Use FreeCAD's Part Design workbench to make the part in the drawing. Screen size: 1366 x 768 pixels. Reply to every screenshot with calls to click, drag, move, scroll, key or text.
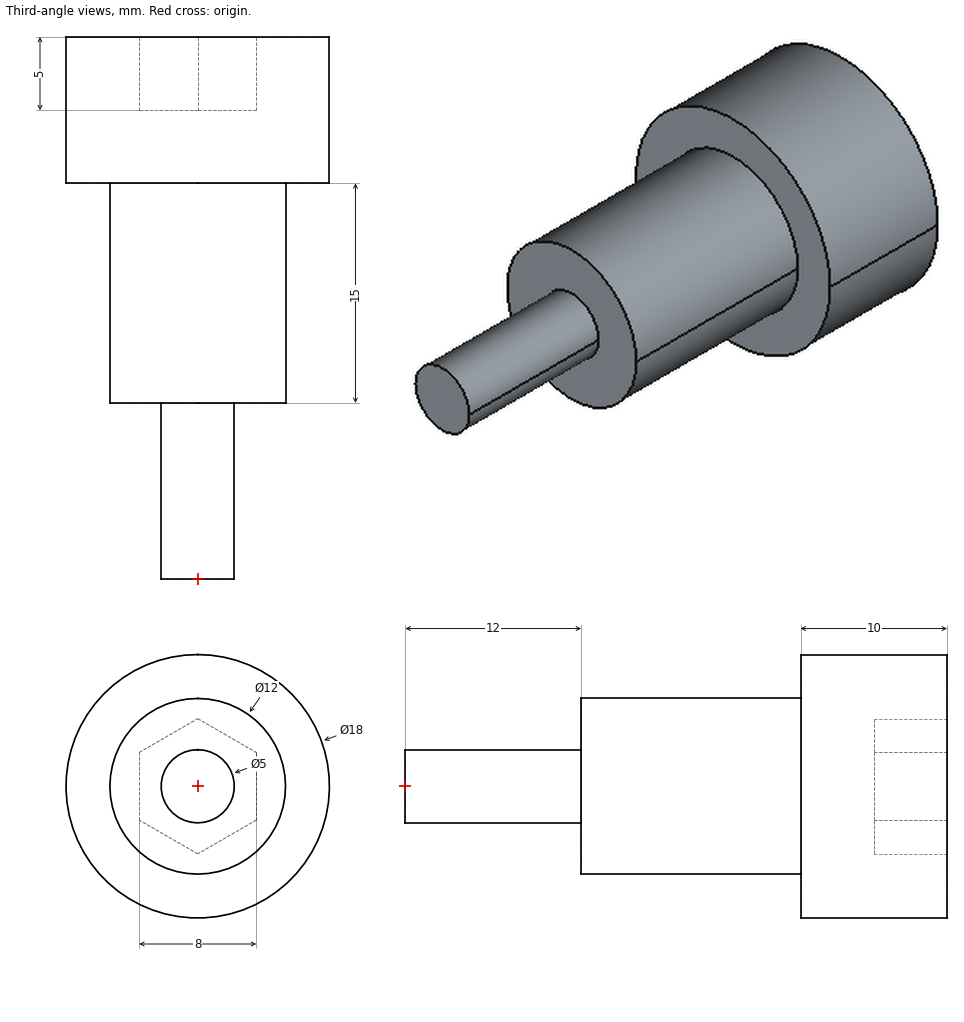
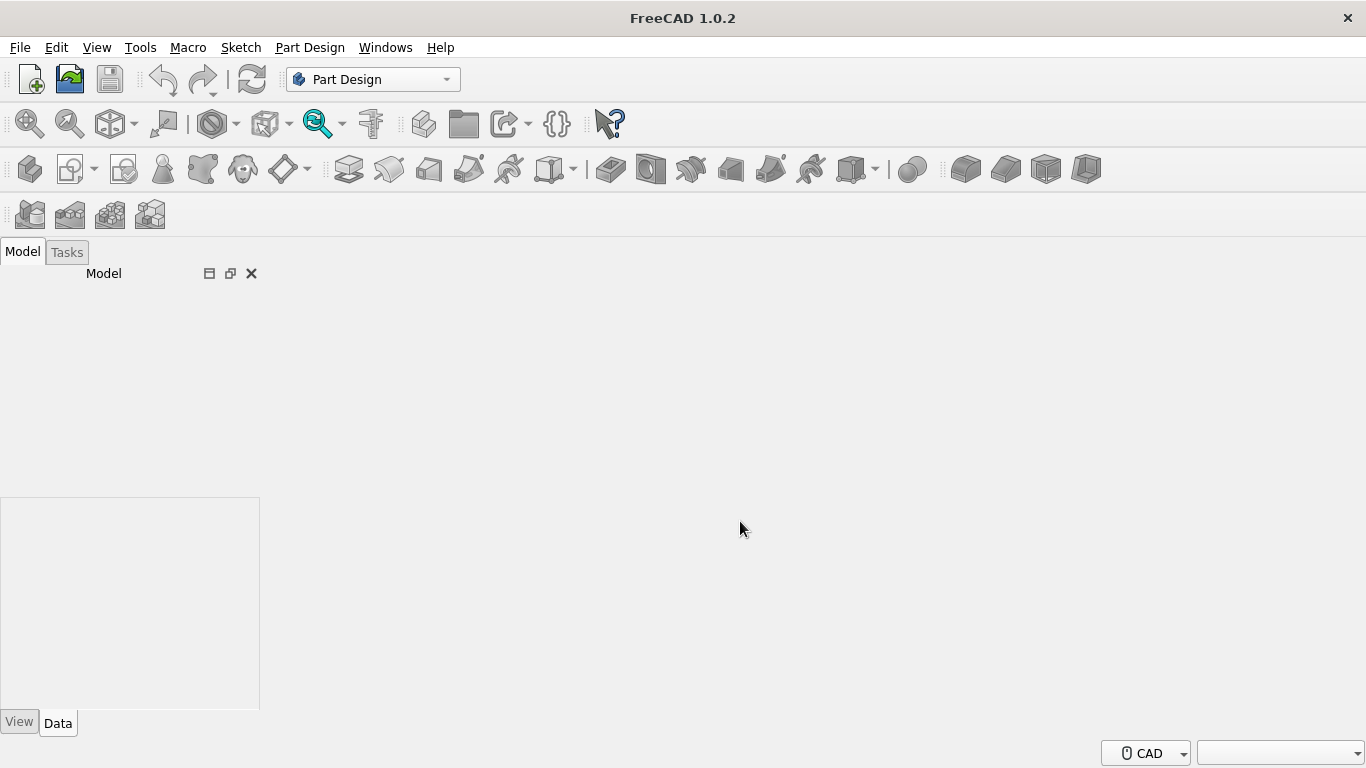
click(30, 80)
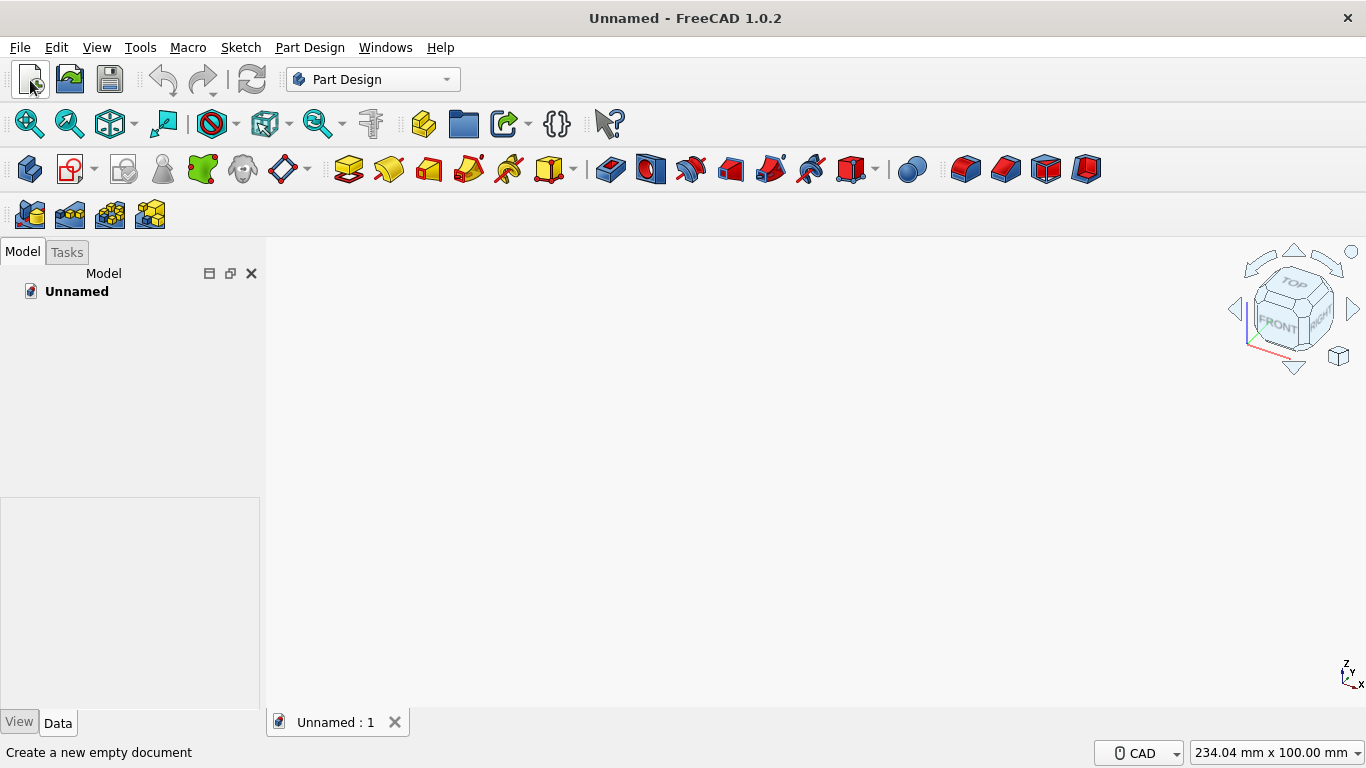
click(70, 170)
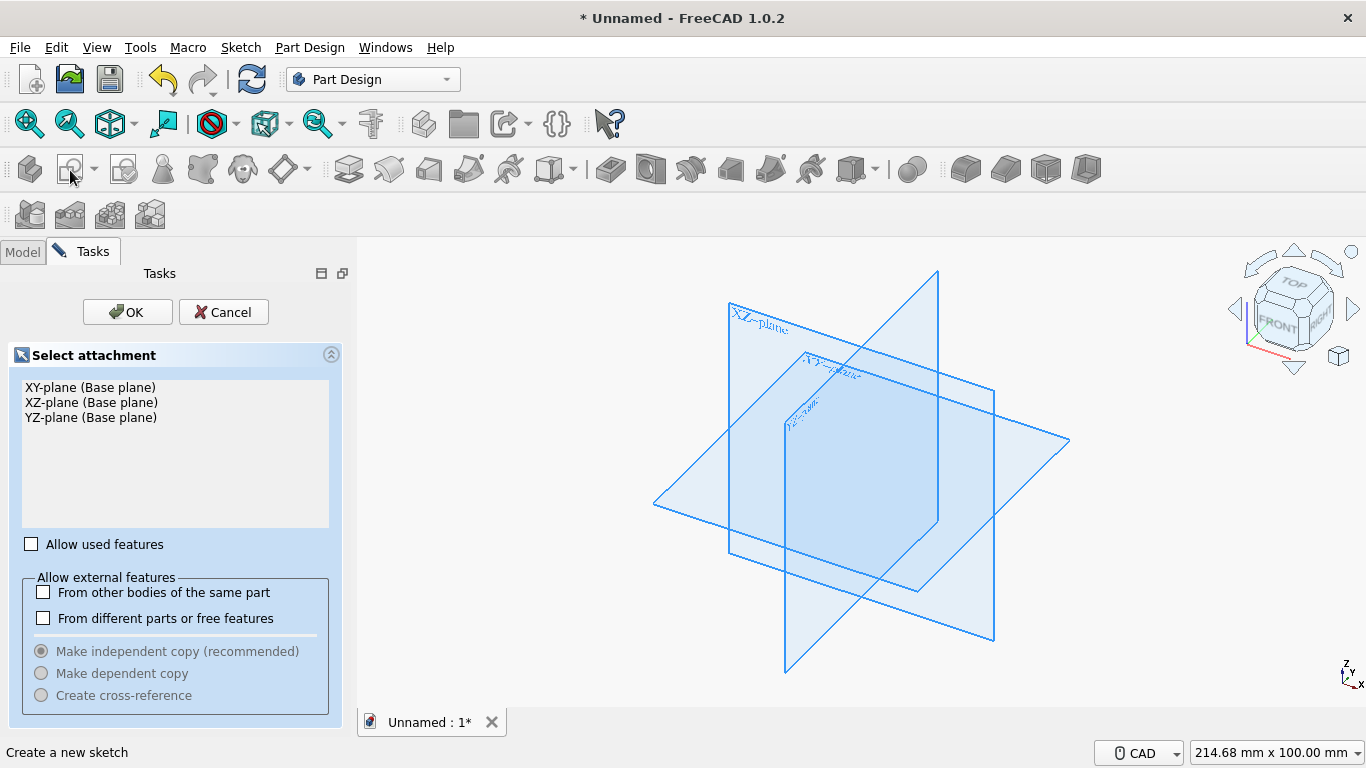
click(82, 402)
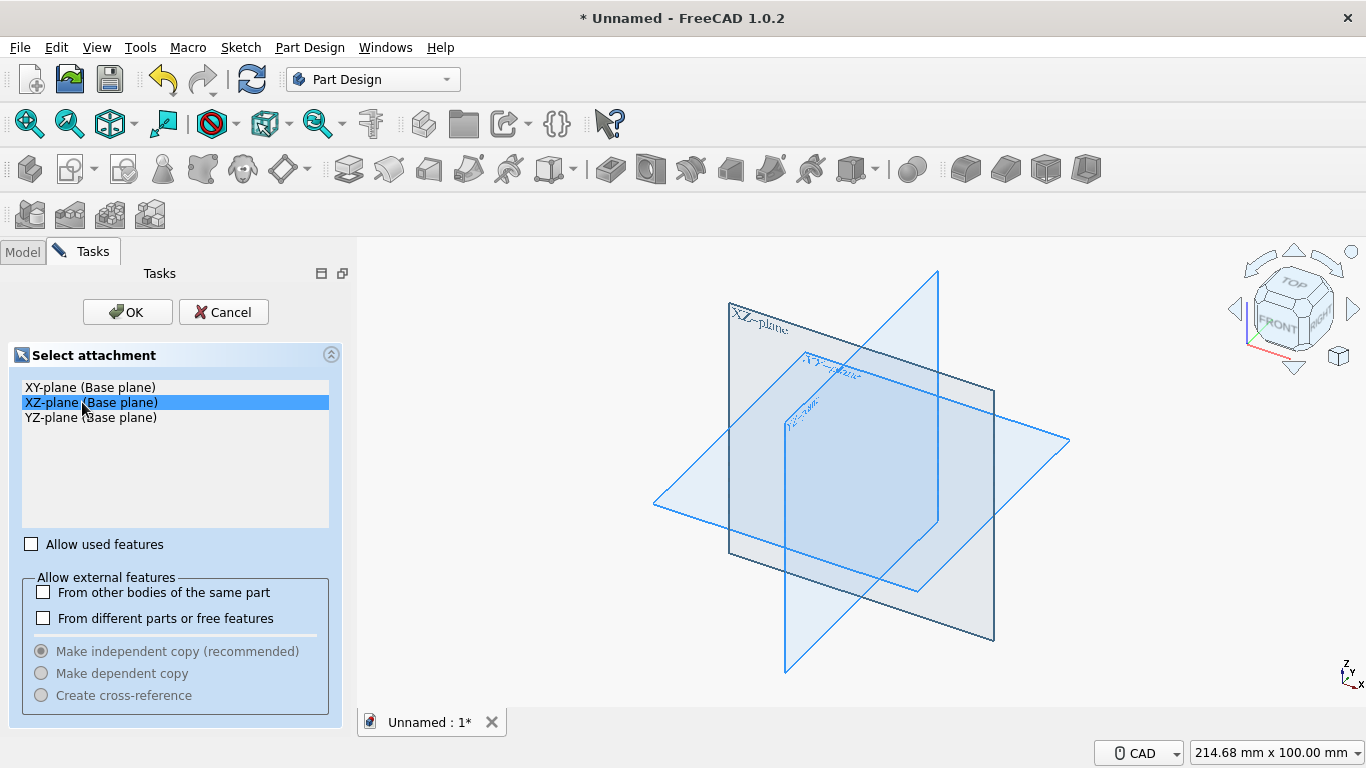
click(128, 312)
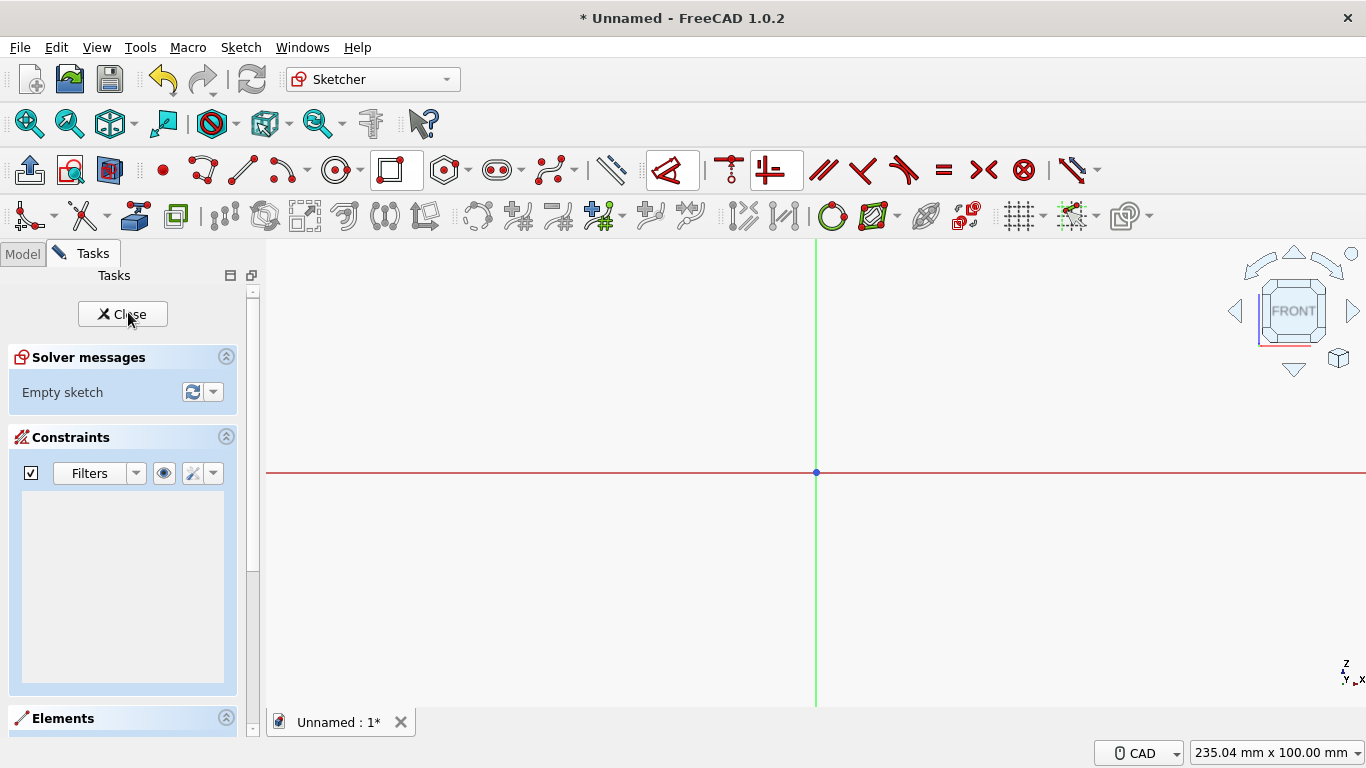
scroll(821, 473, up, 13)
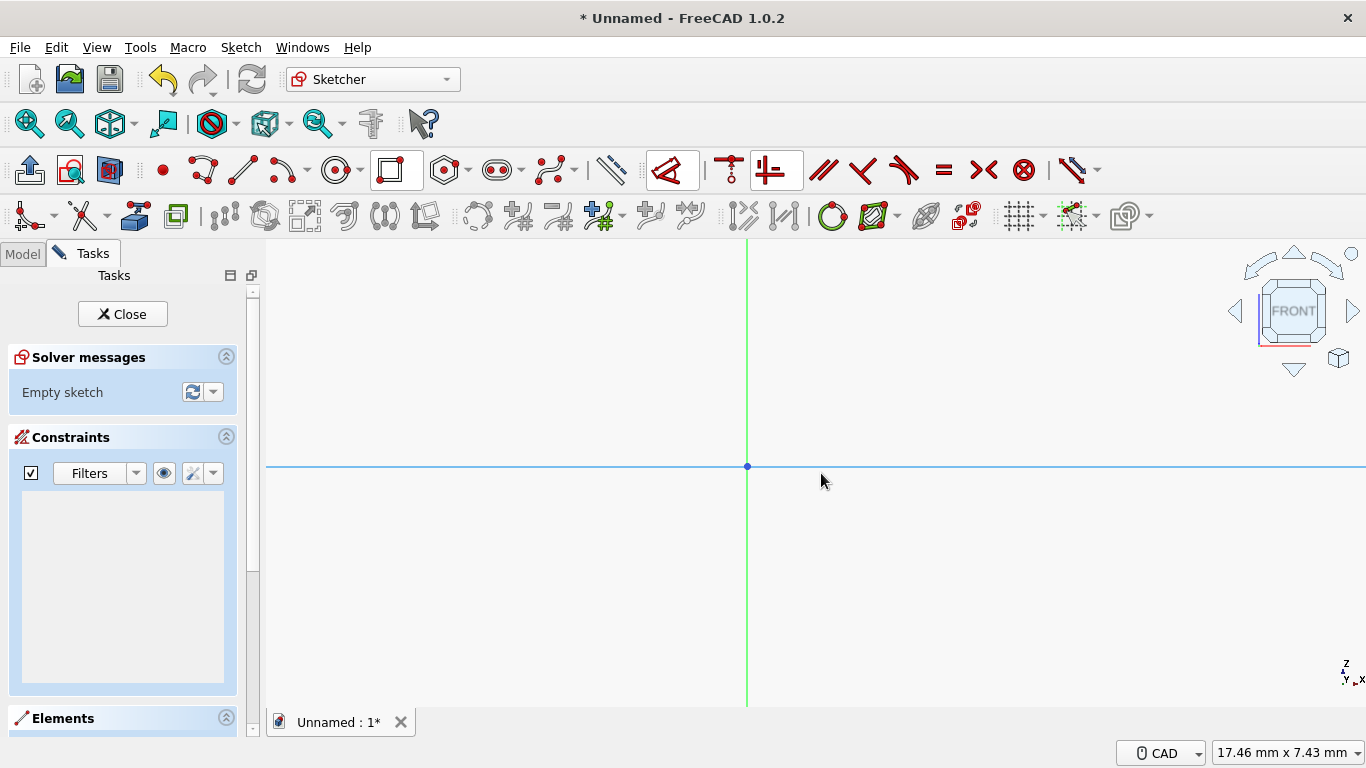
click(336, 170)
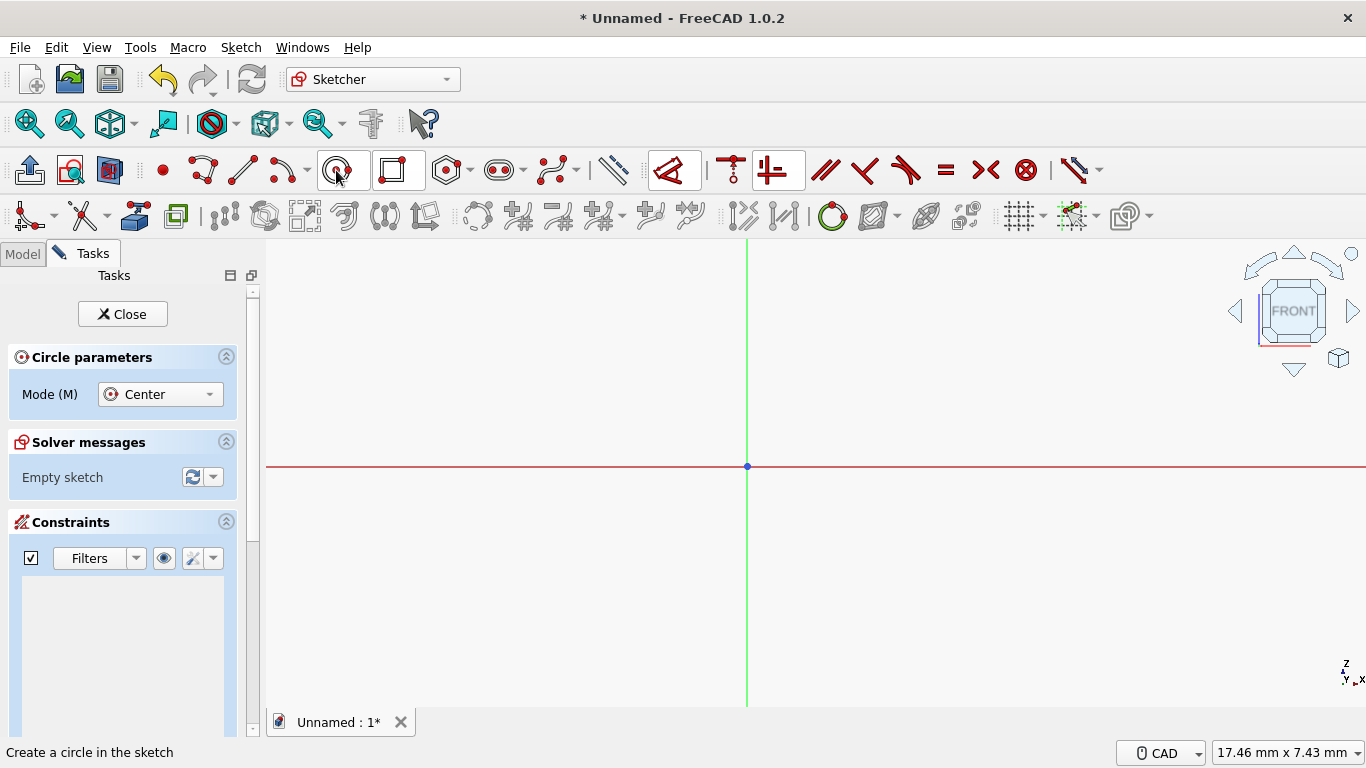
click(747, 467)
move(859, 355)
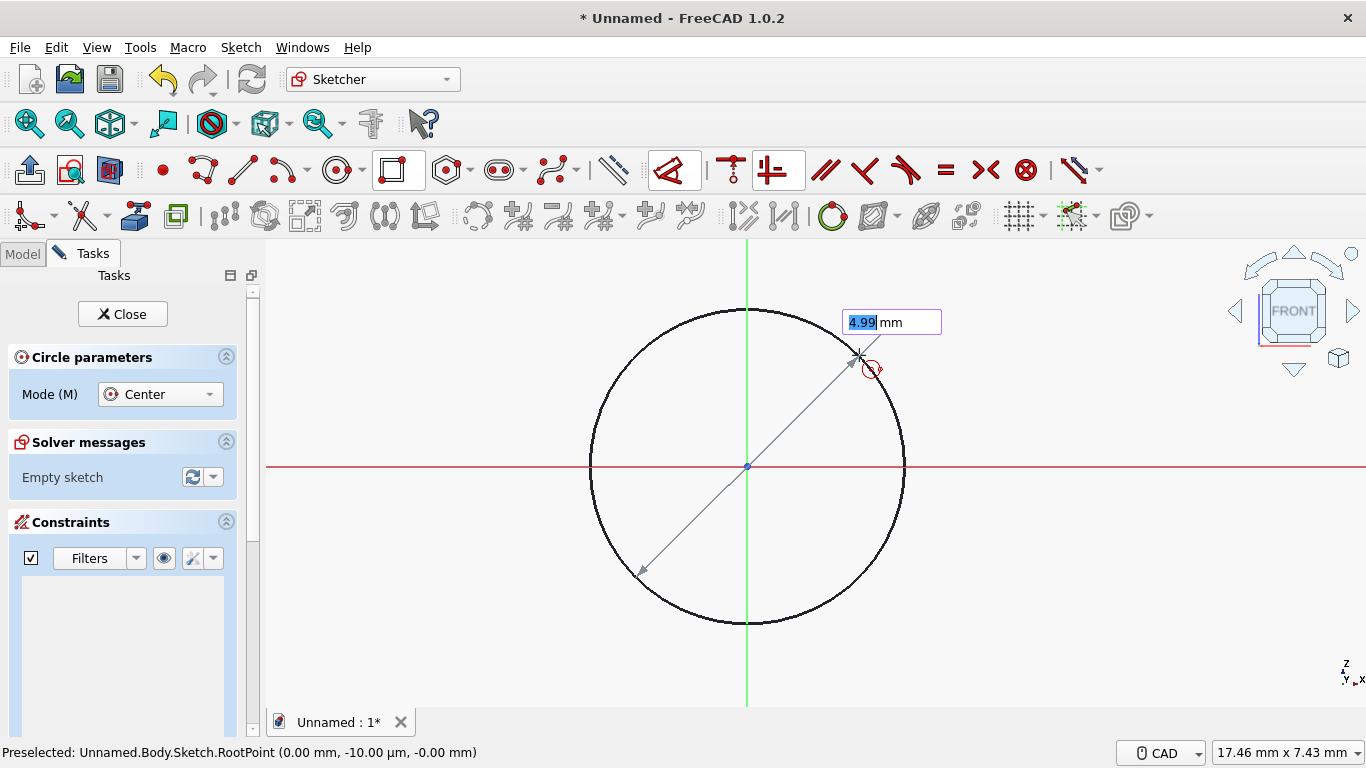
text(5)
key(Return)
key(Escape)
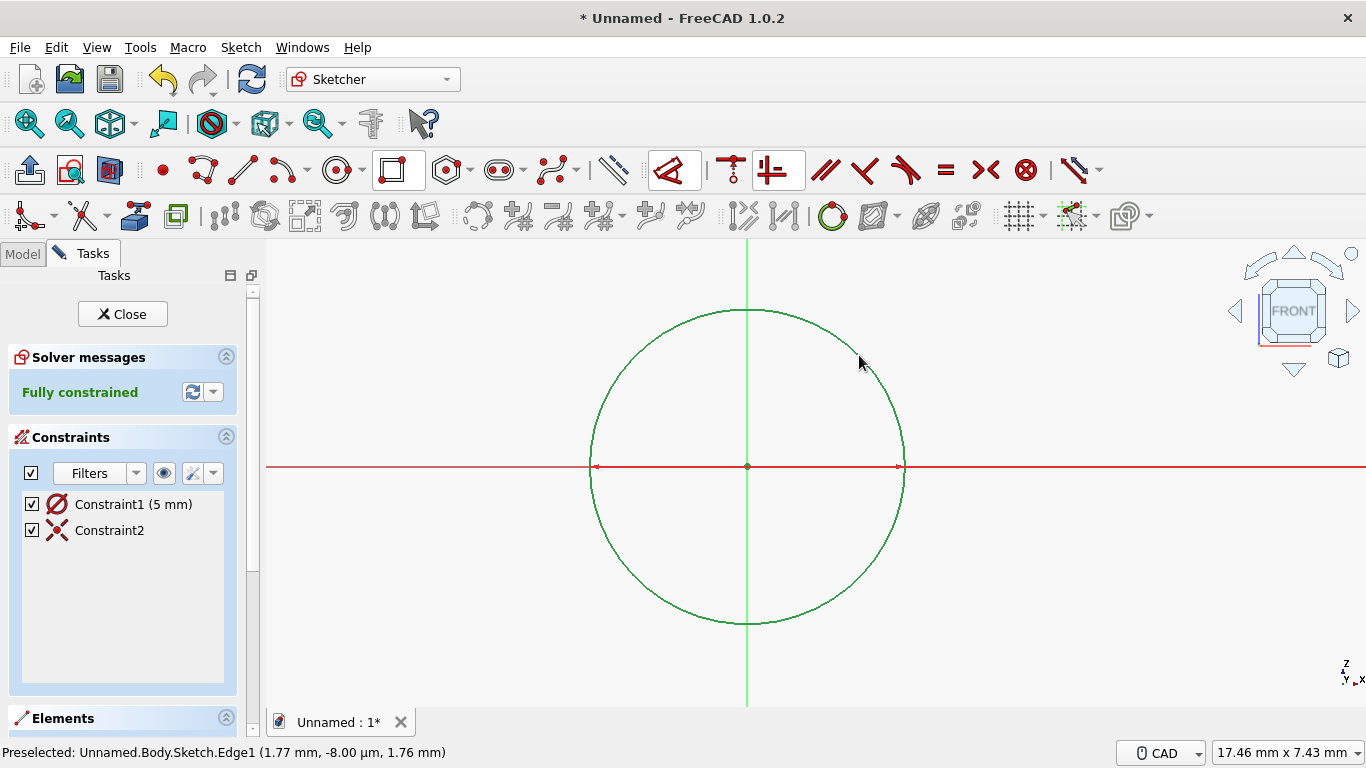
click(123, 314)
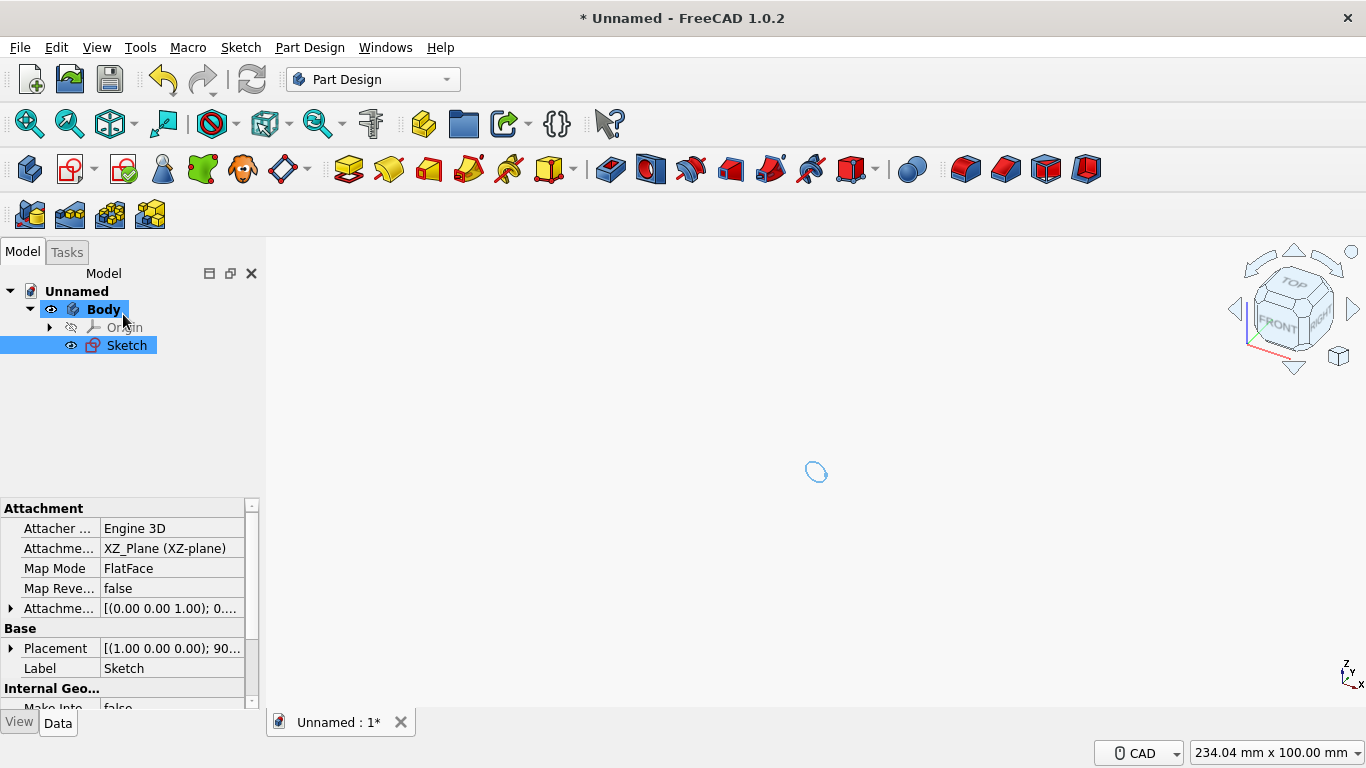
click(350, 170)